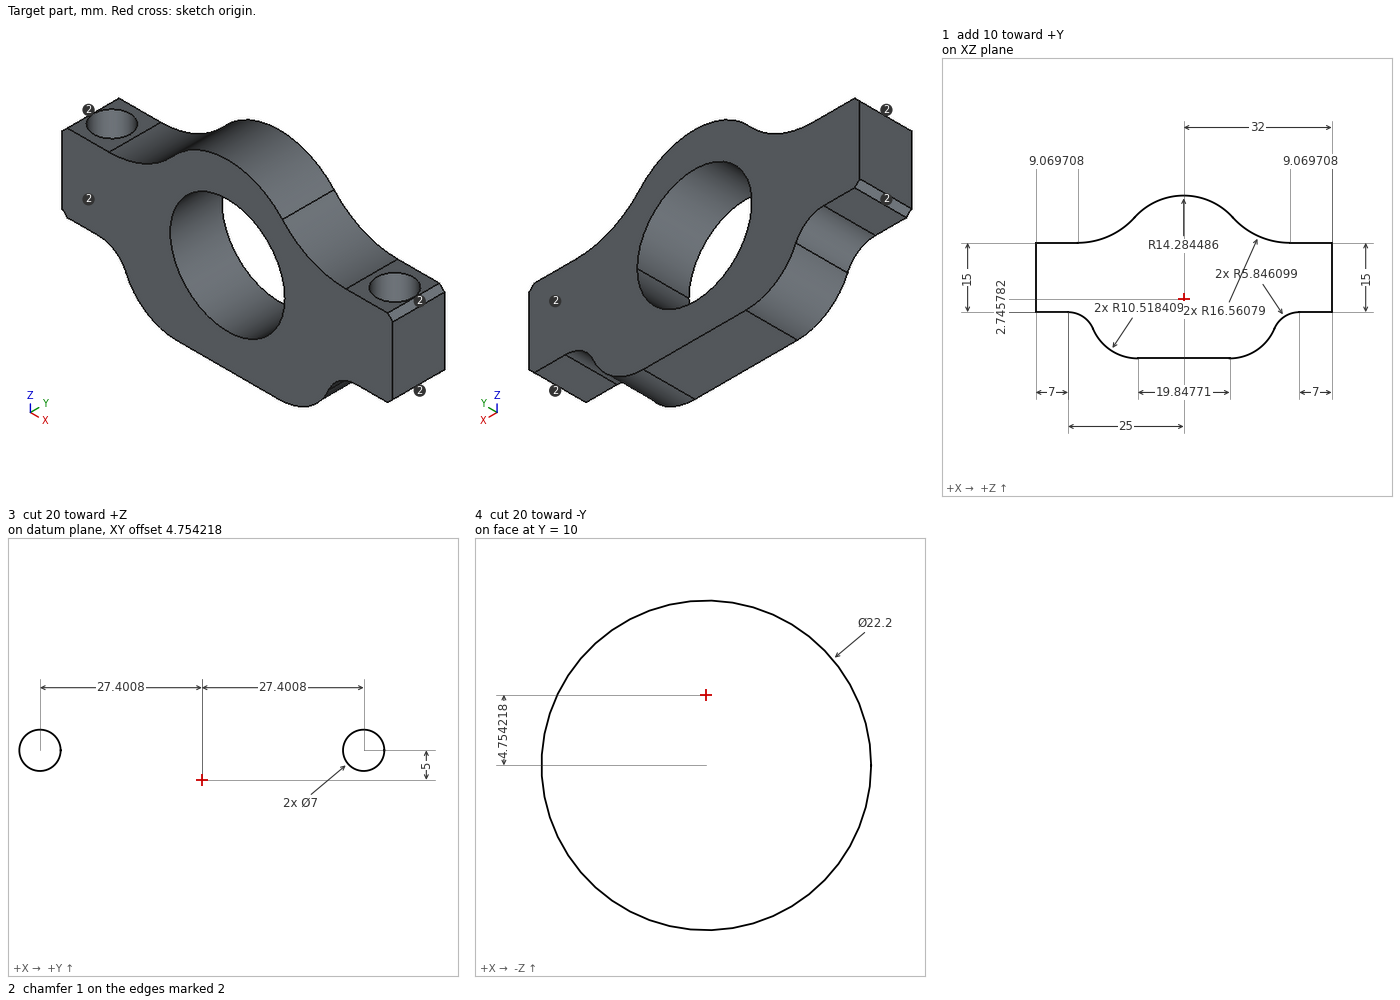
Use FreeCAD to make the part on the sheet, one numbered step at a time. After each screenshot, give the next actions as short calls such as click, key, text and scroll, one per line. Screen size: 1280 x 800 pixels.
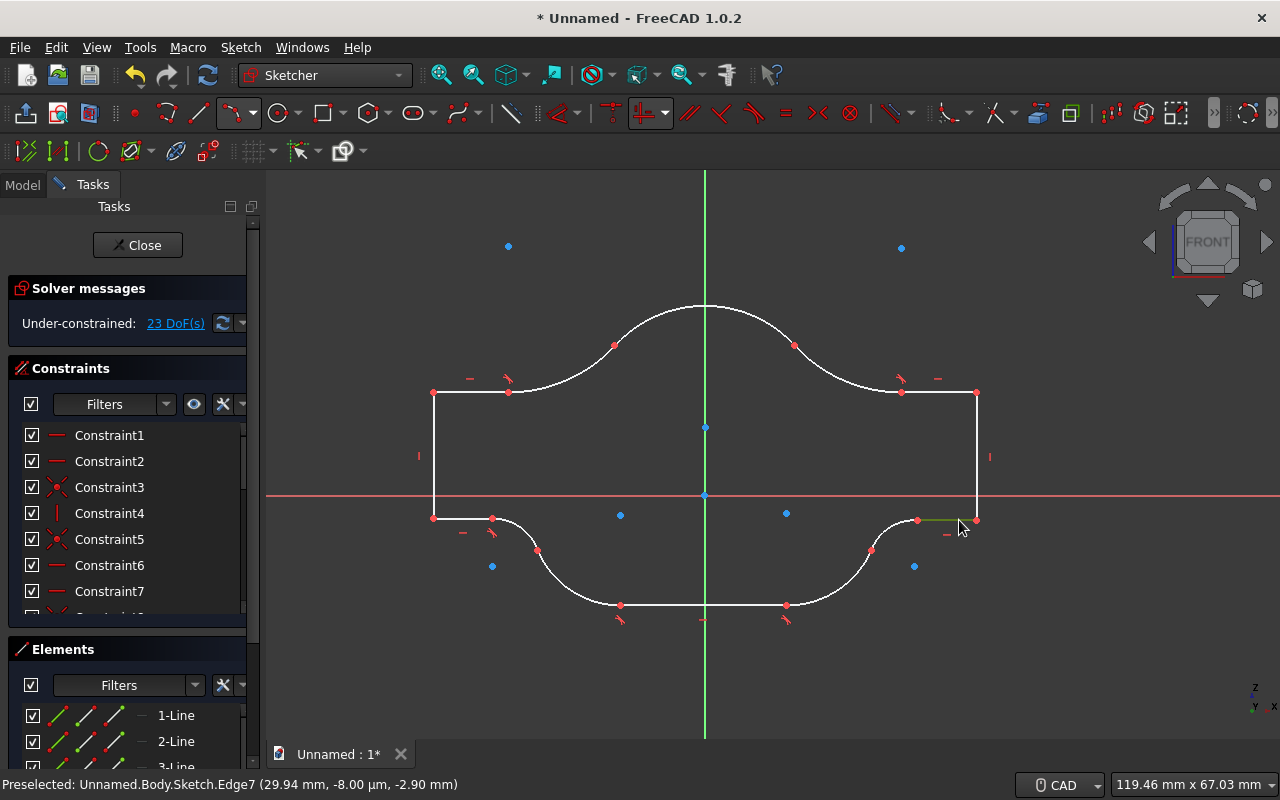
click(900, 523)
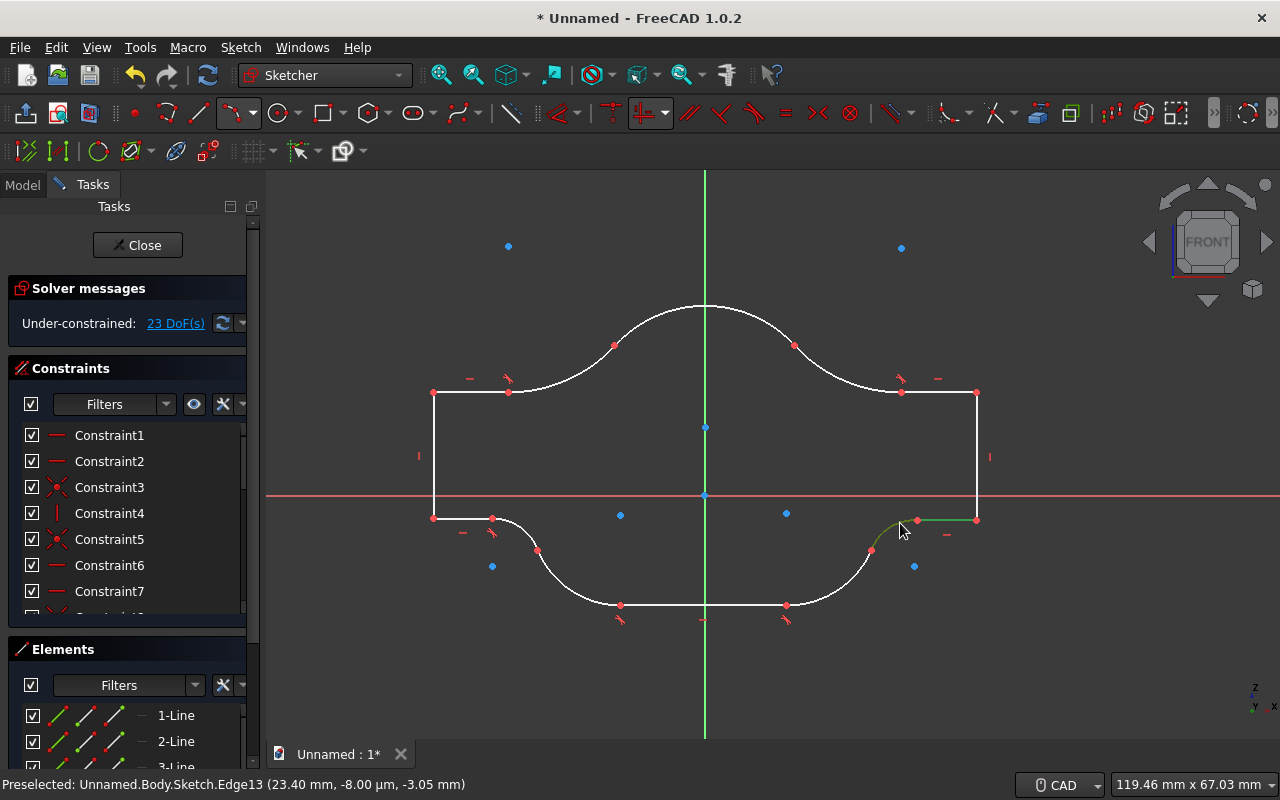
click(754, 114)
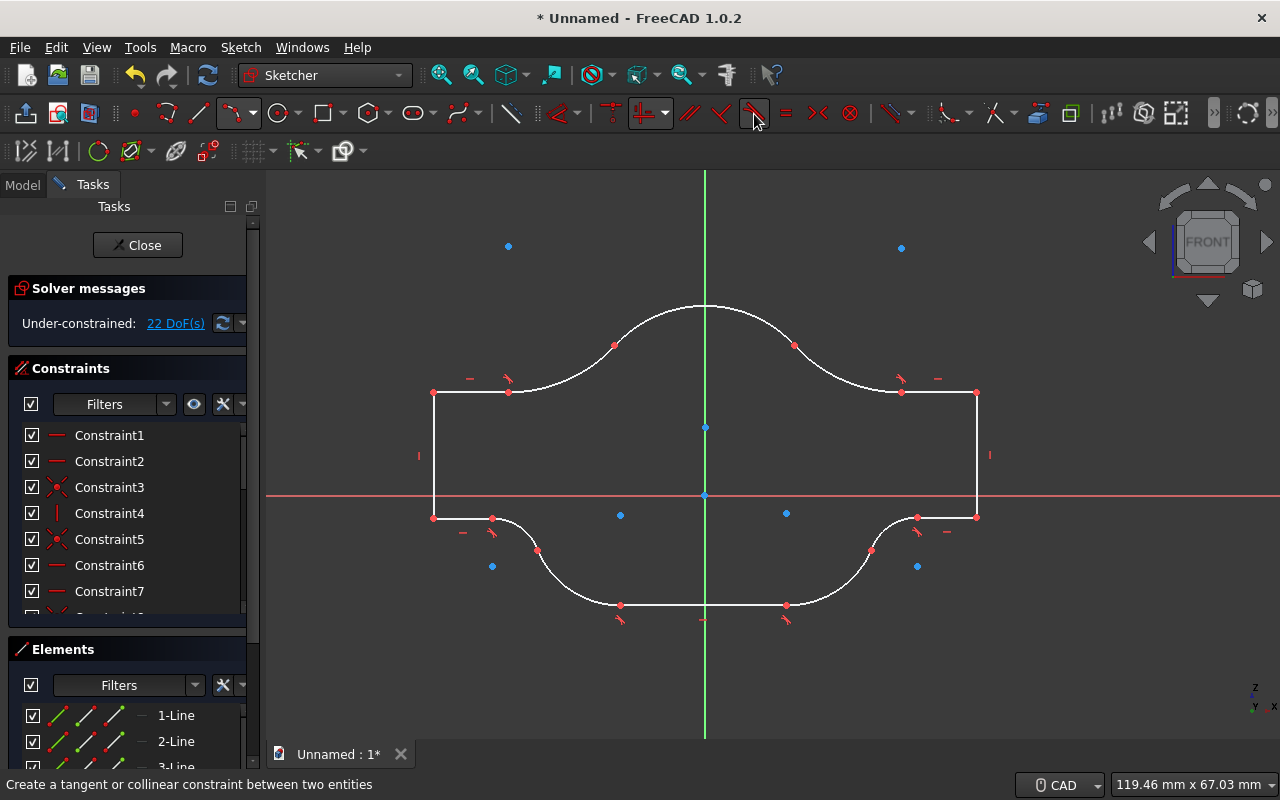
click(555, 577)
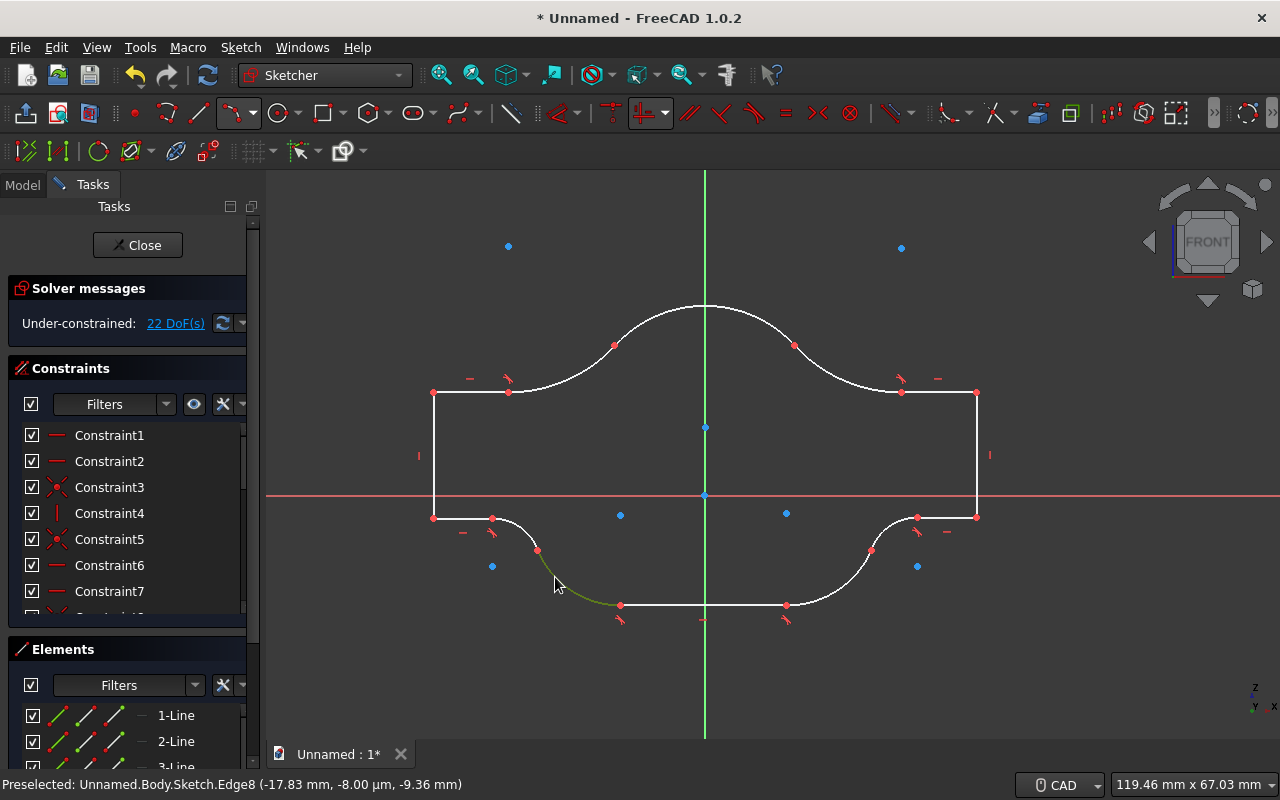
click(529, 535)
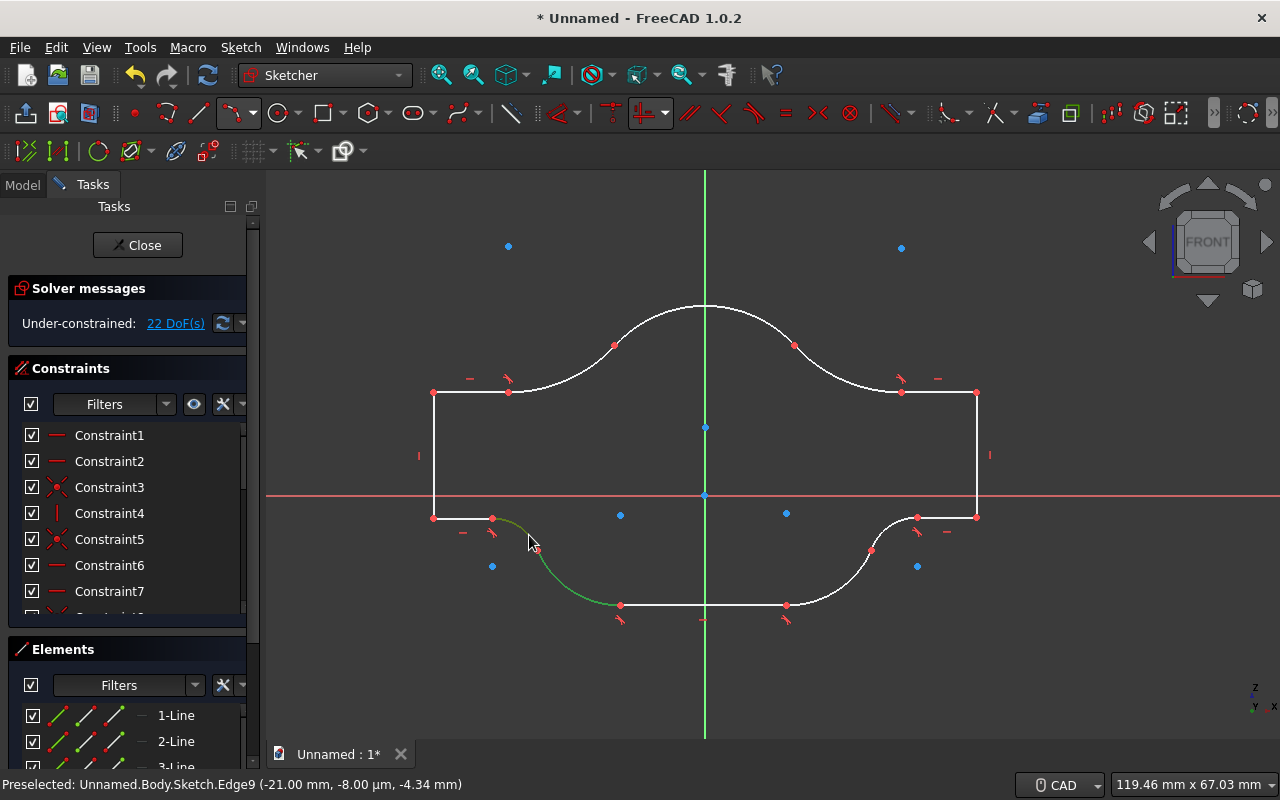
click(754, 114)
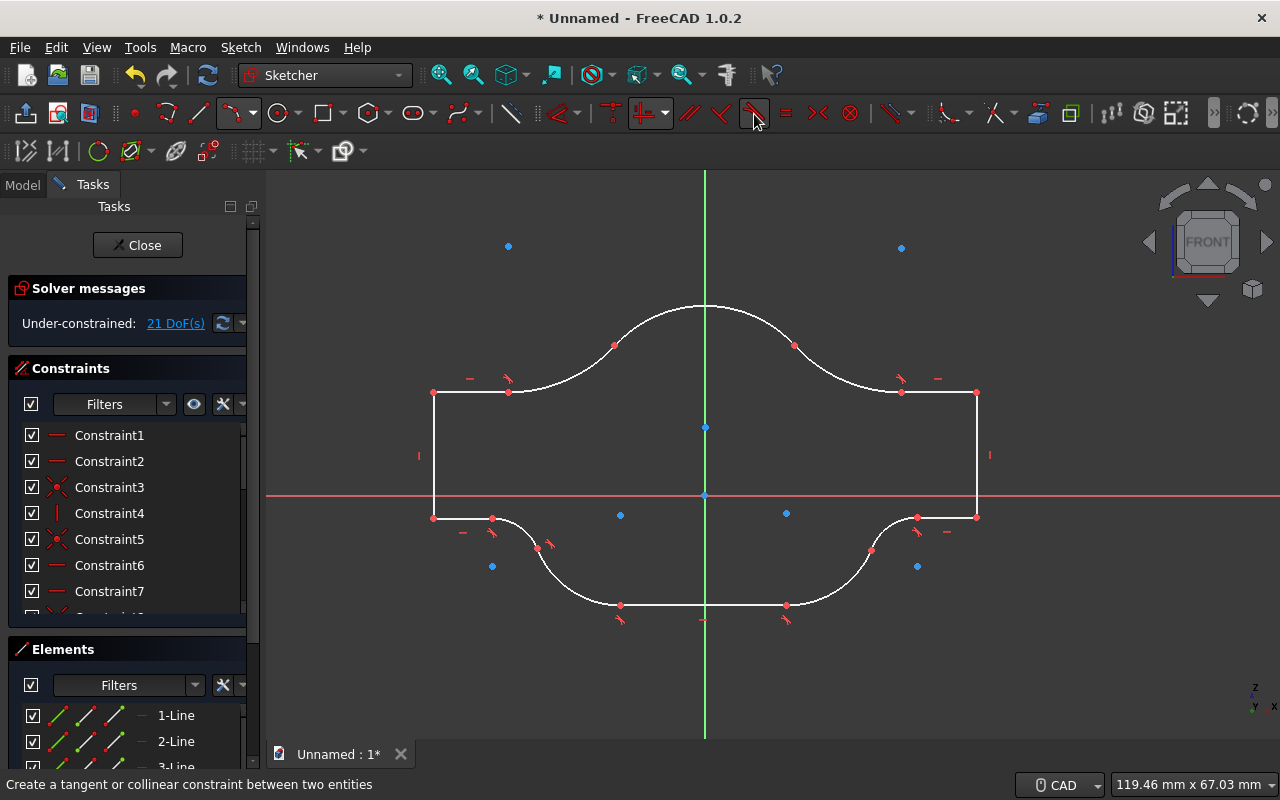
click(544, 388)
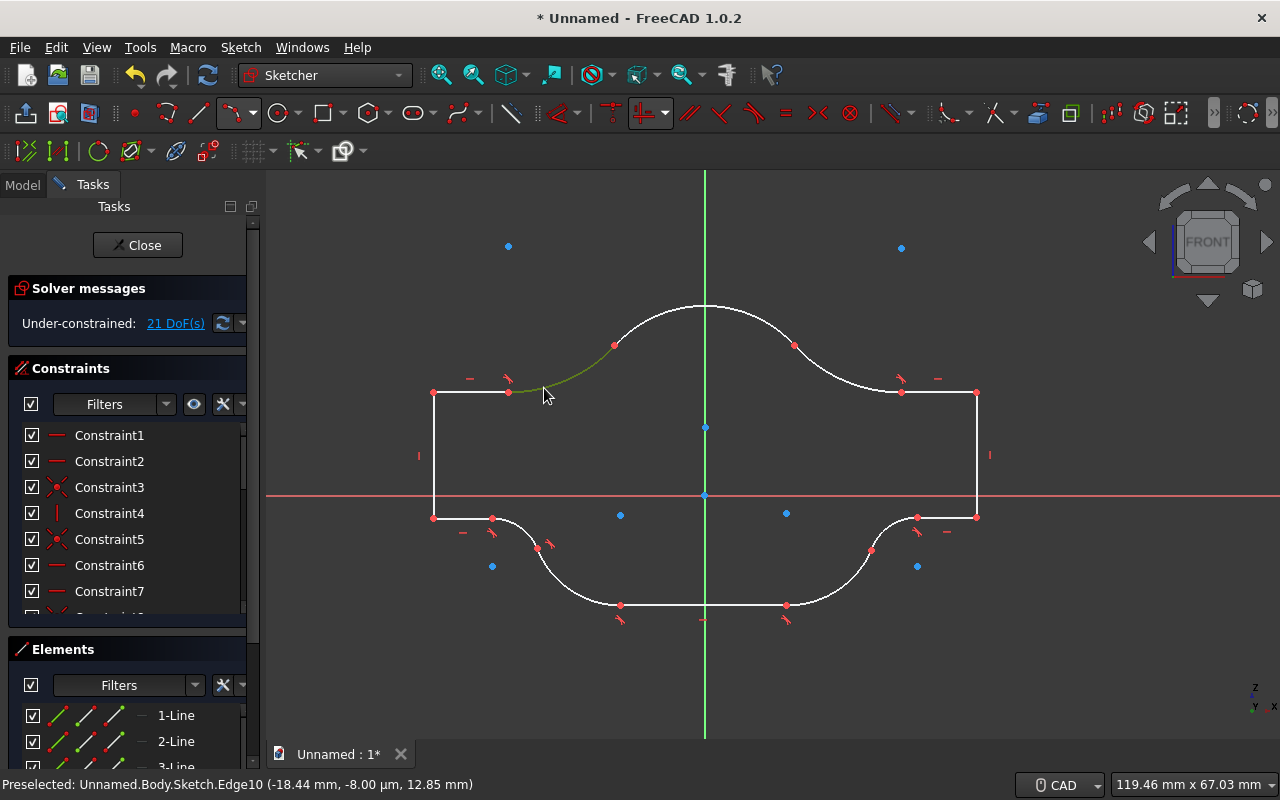
click(745, 313)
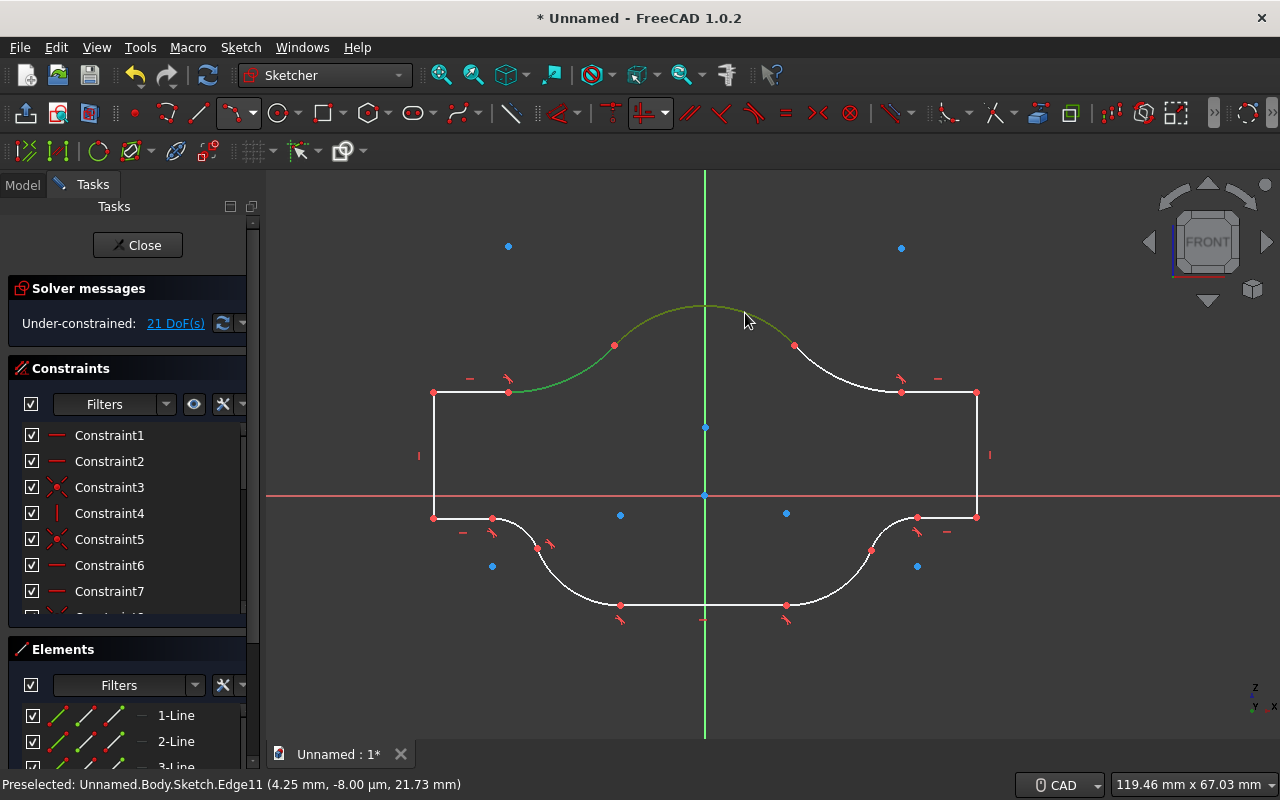
click(754, 114)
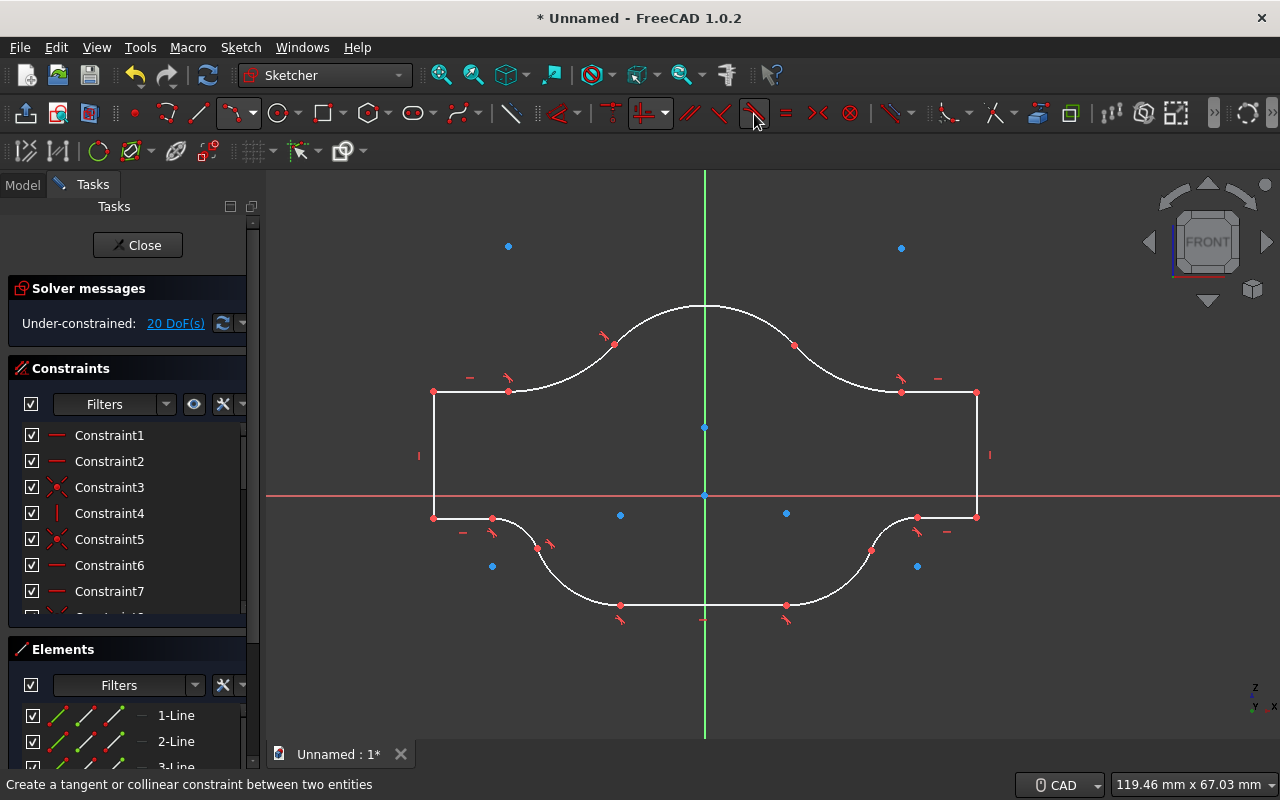
click(745, 312)